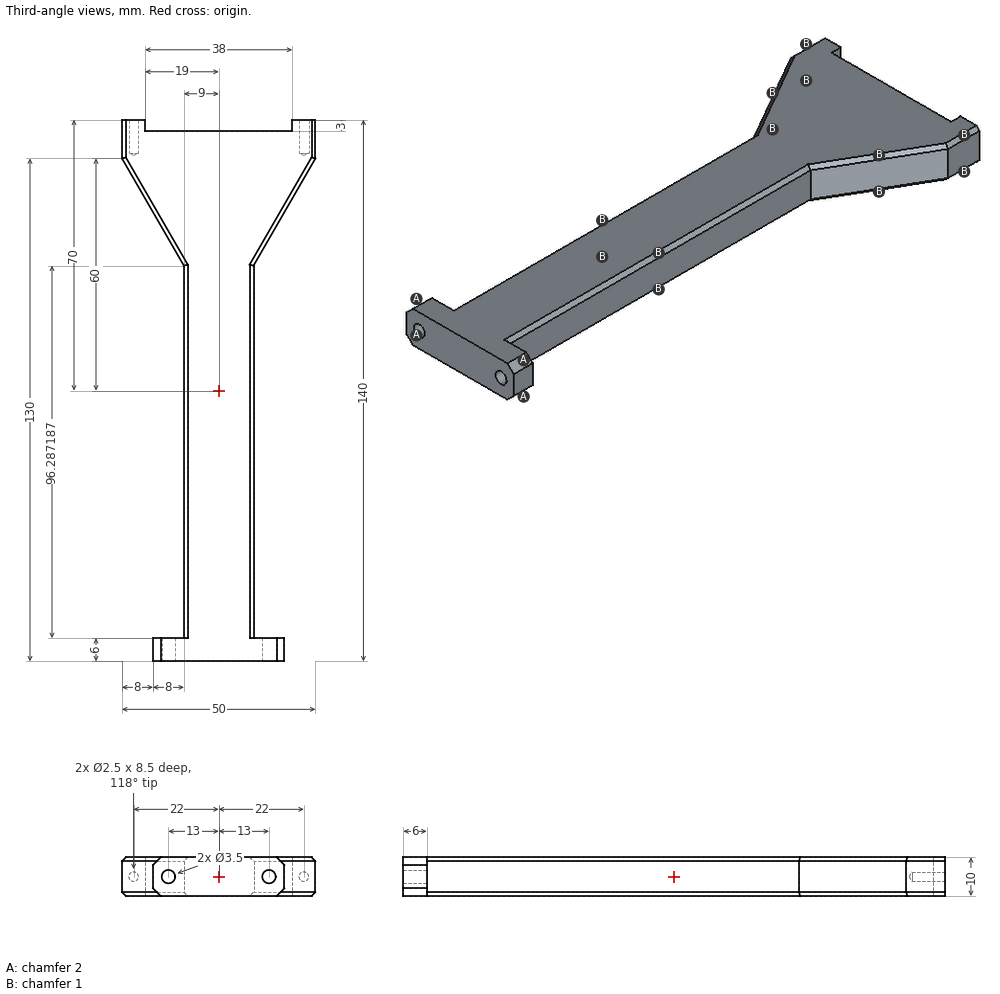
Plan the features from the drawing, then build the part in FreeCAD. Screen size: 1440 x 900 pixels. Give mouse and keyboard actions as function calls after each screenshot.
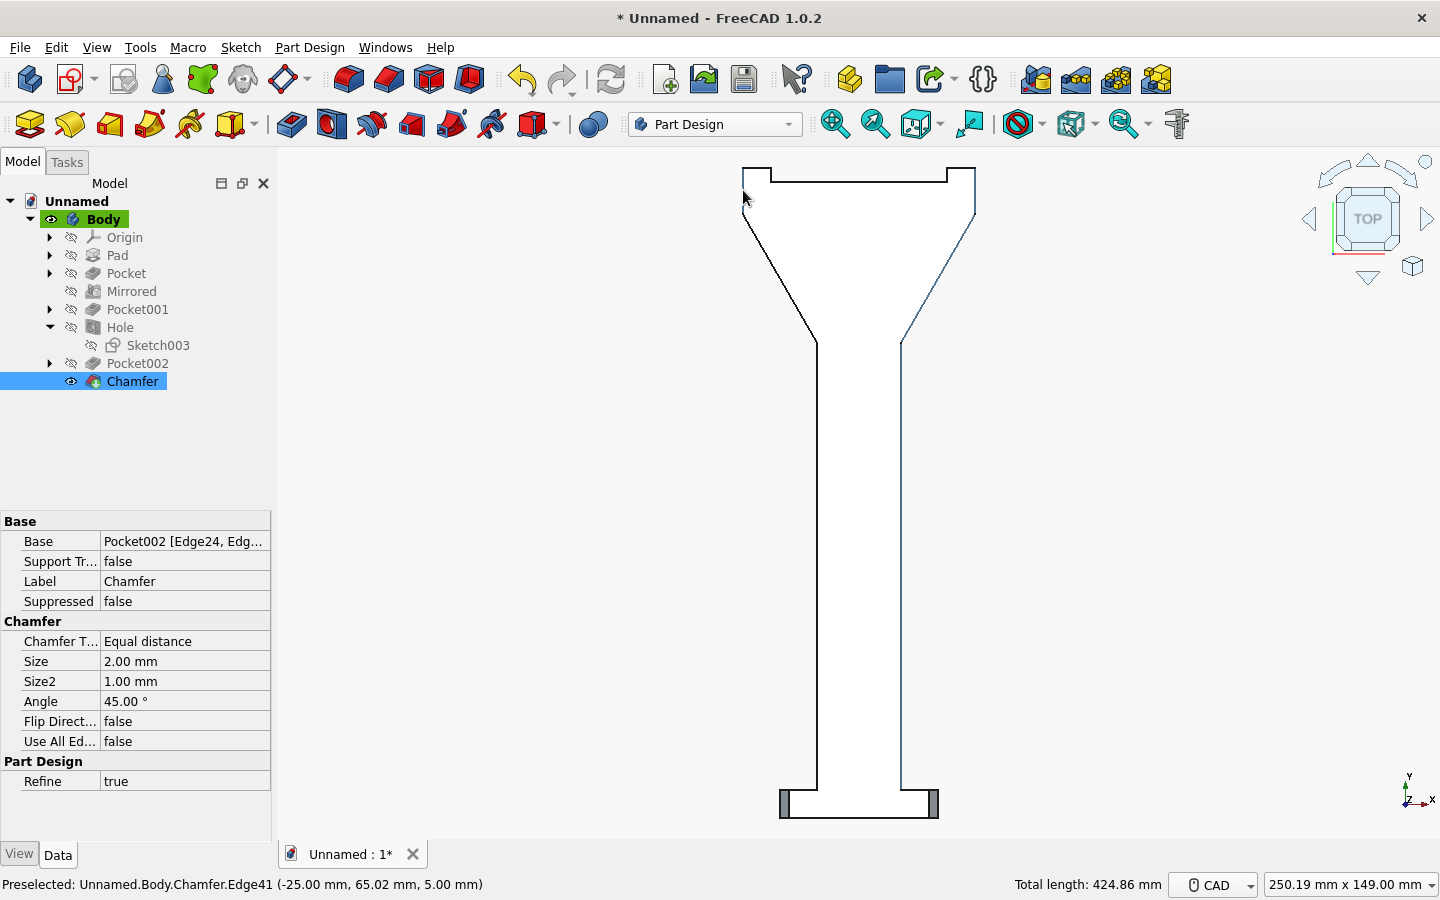
click(817, 566, ctrl)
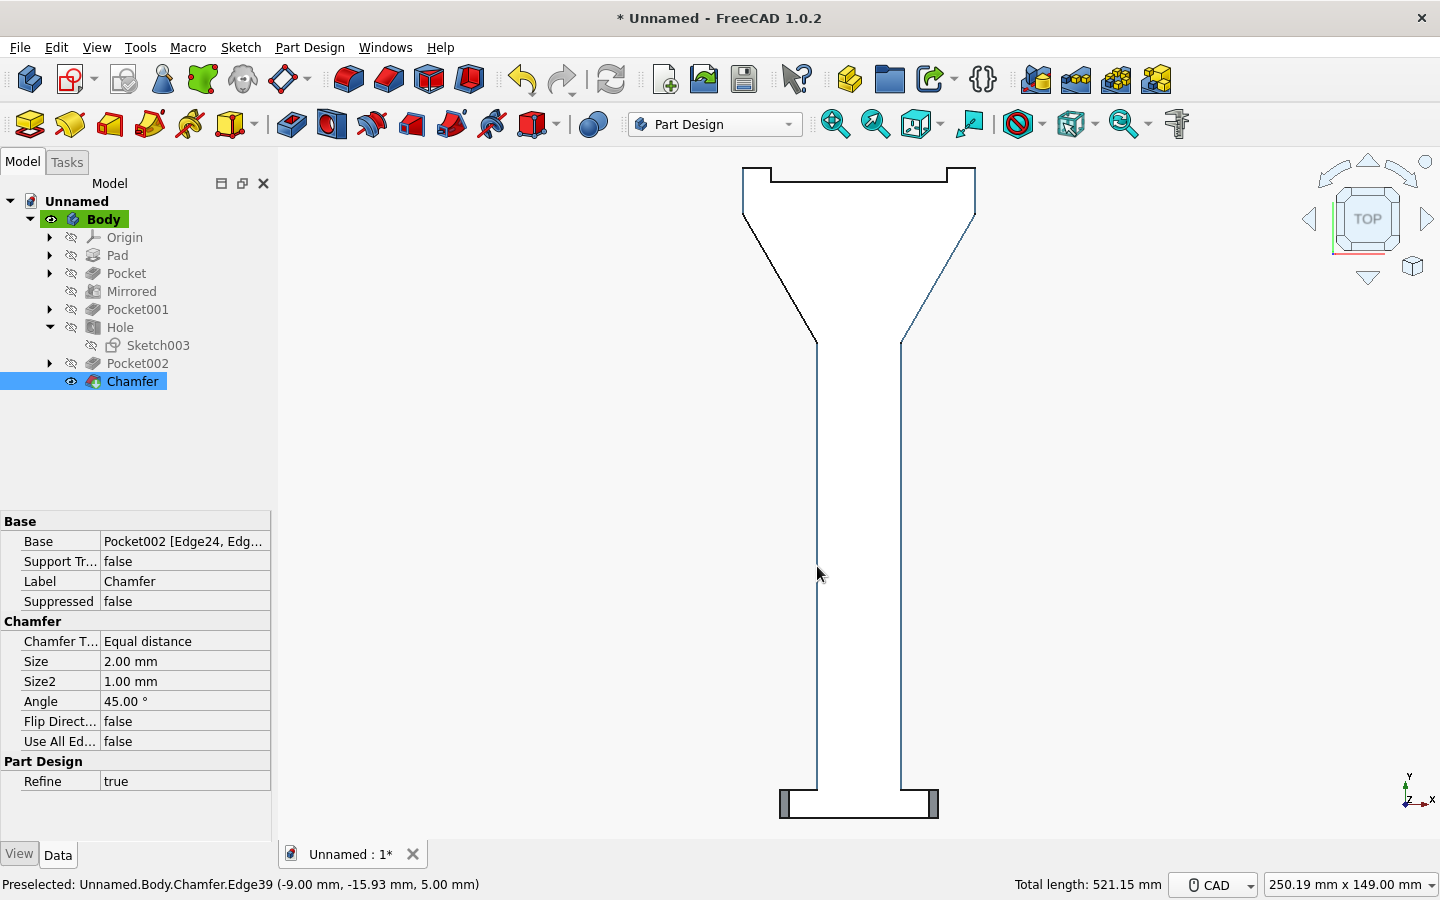
click(780, 278, ctrl)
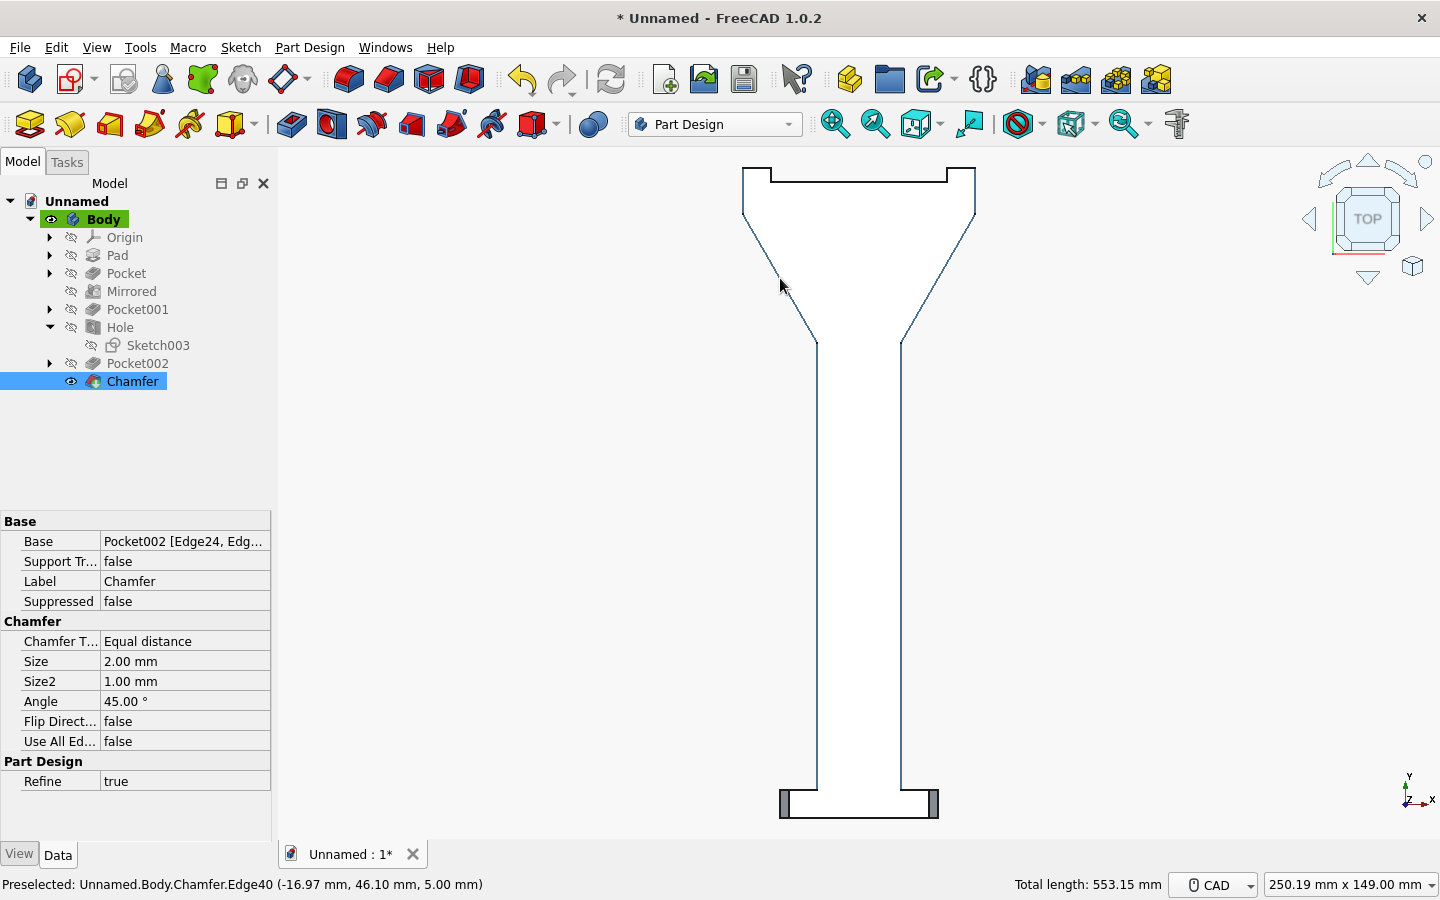
click(390, 80)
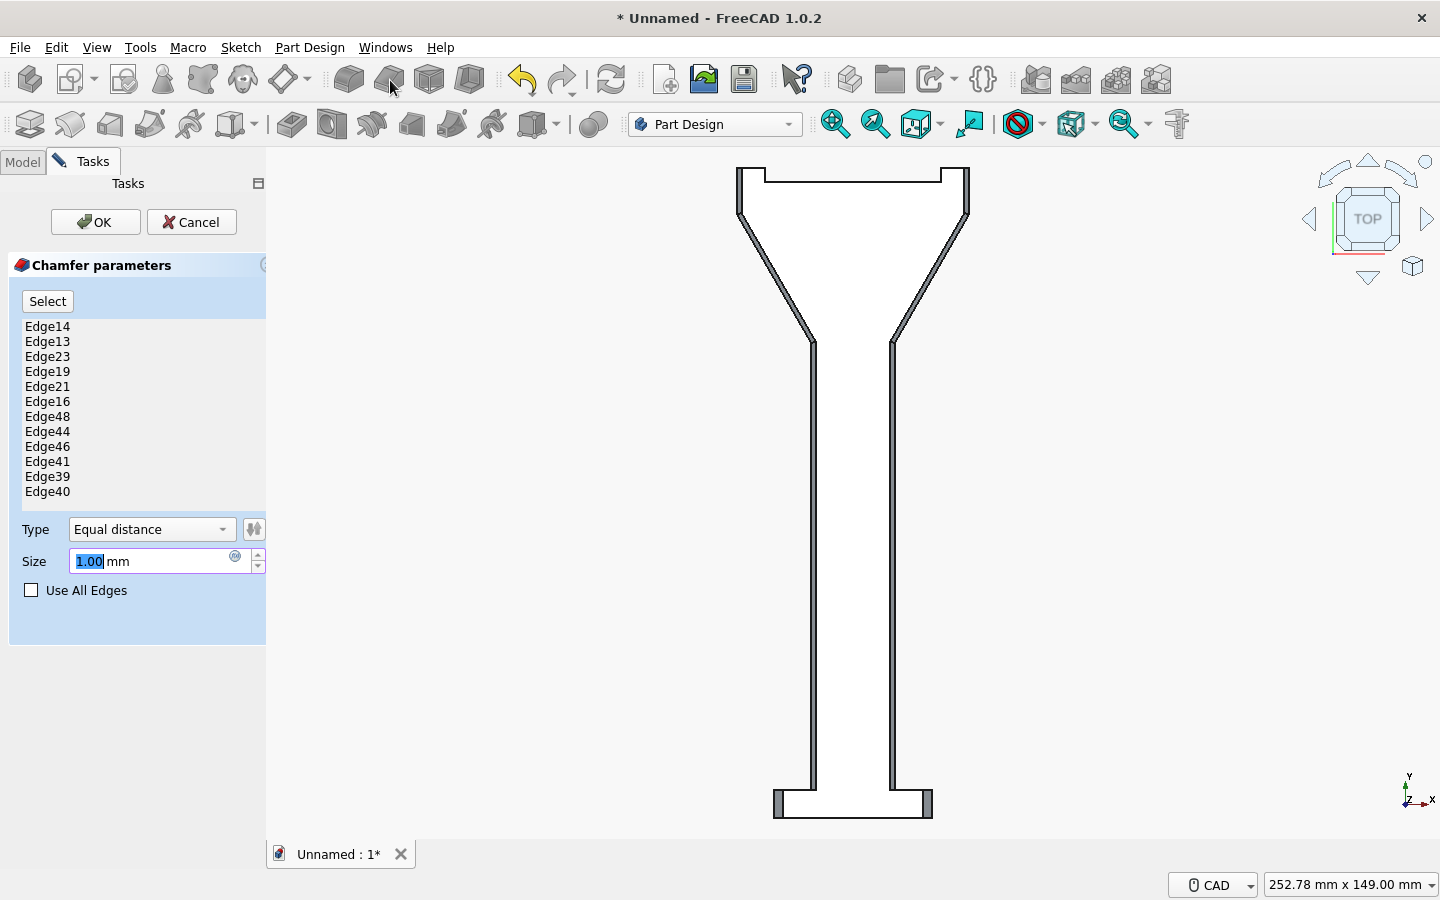
text(1)
key(Tab)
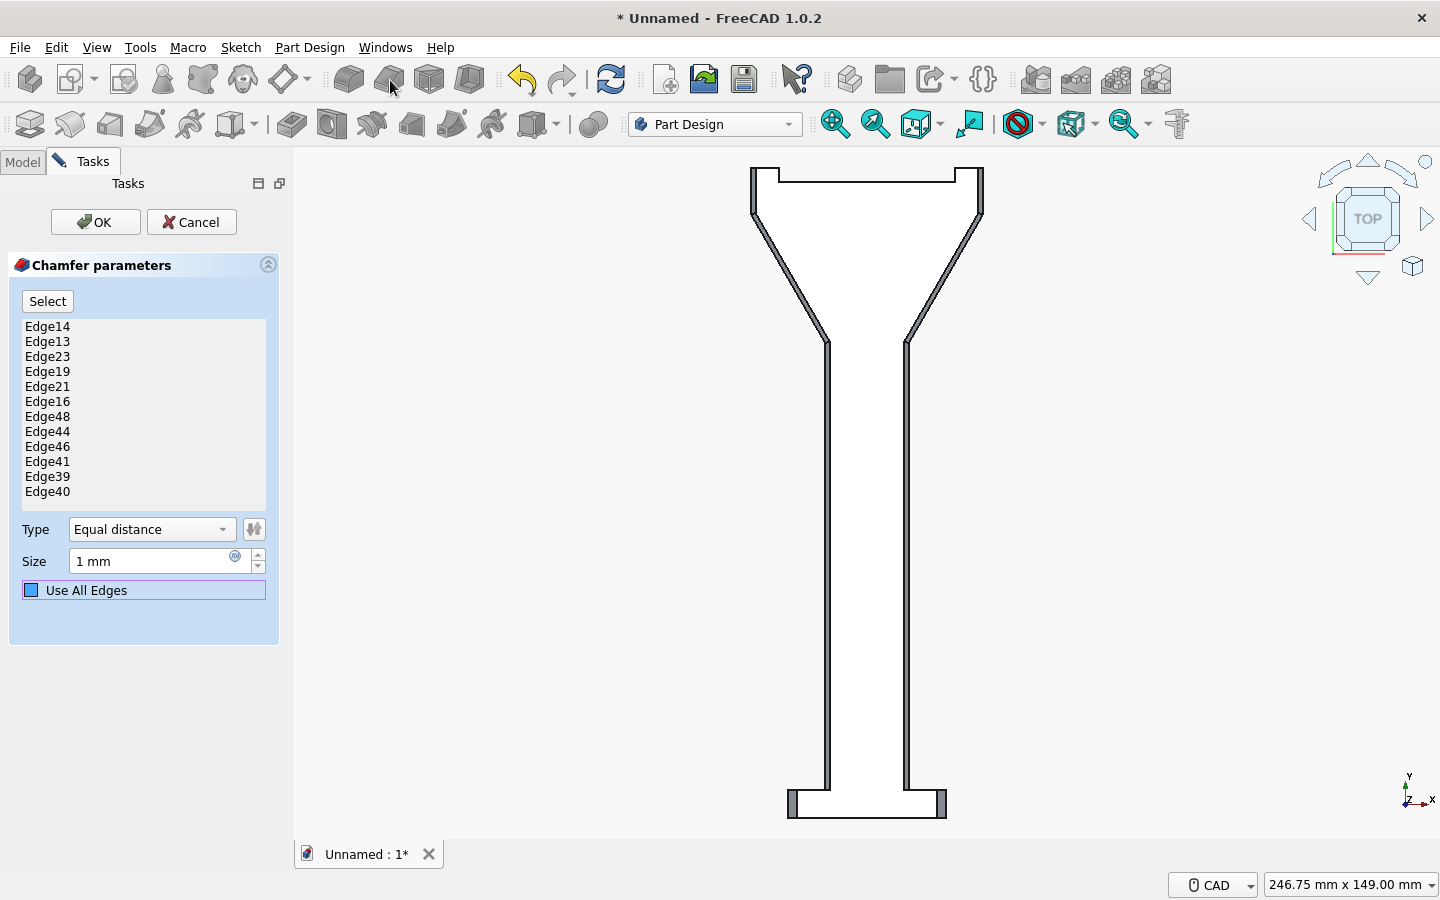
click(96, 222)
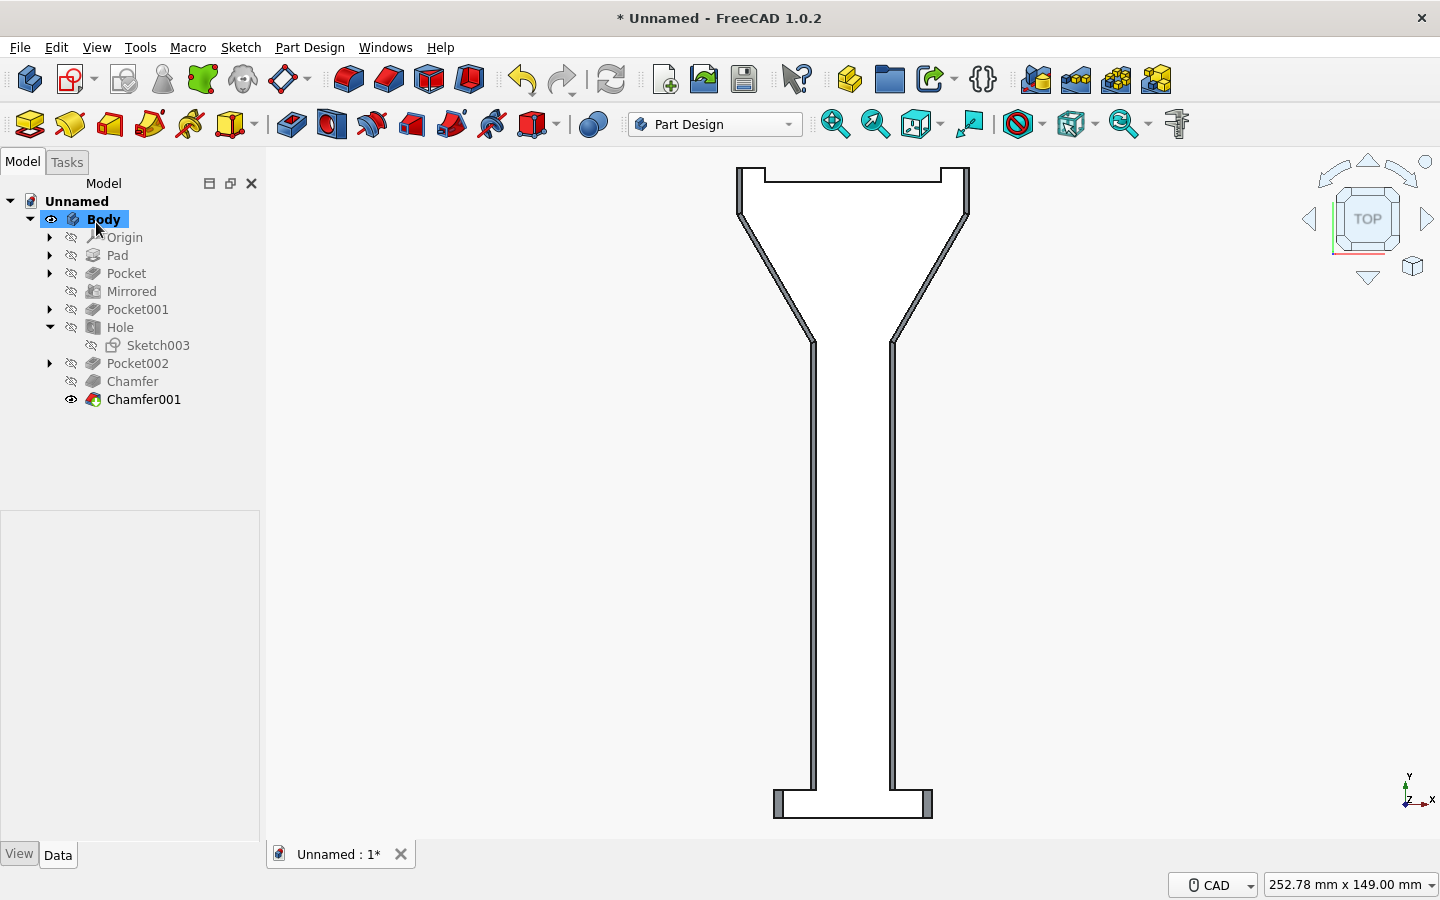
key(0)